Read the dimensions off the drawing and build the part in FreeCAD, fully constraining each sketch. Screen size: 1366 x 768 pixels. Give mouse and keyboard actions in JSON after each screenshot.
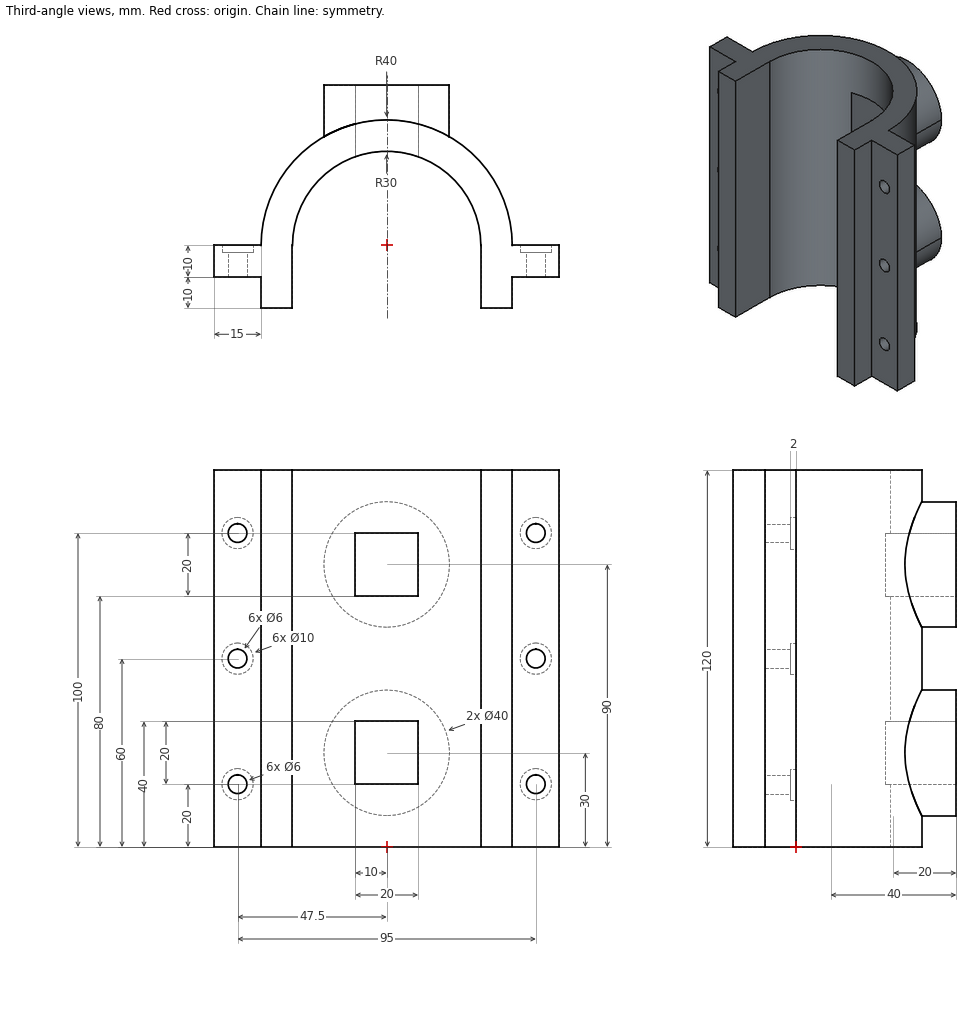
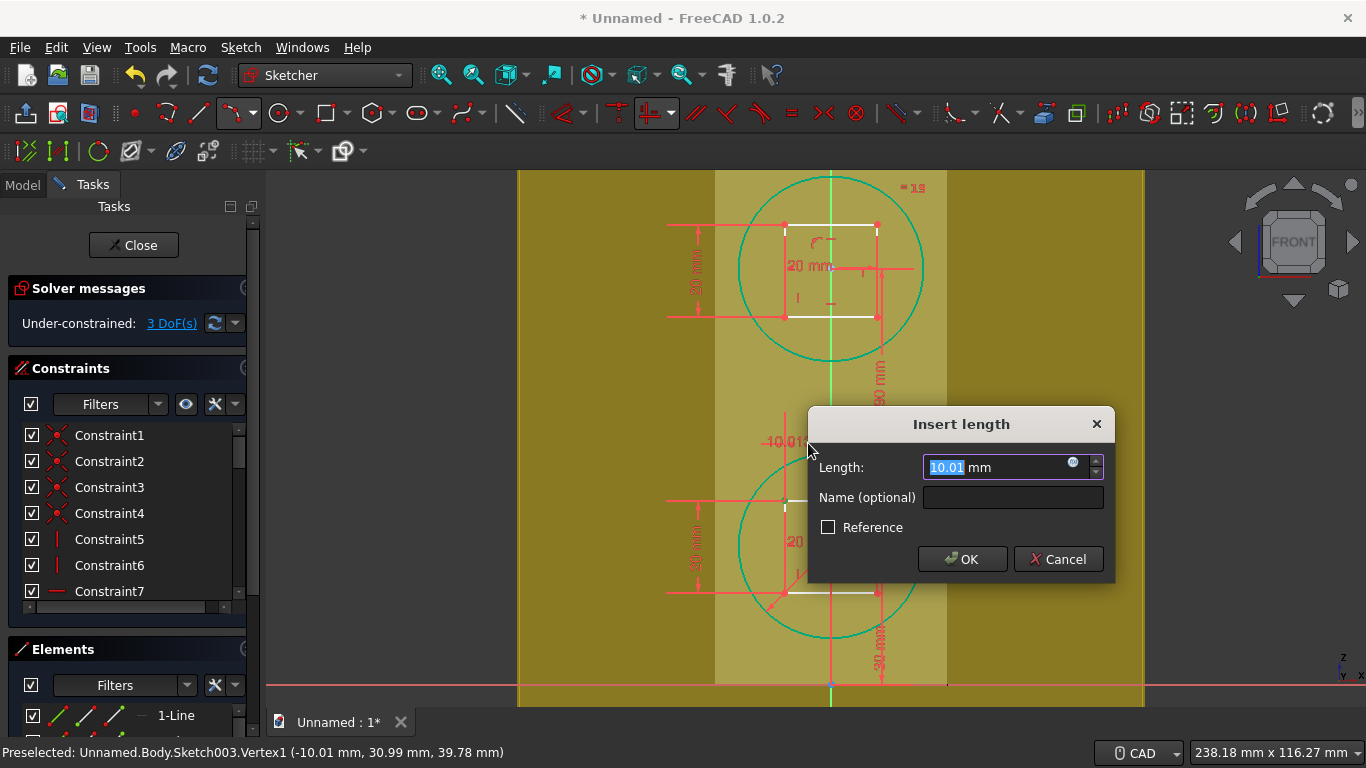
{"action": "type", "text": "10"}
{"action": "key", "text": "Return"}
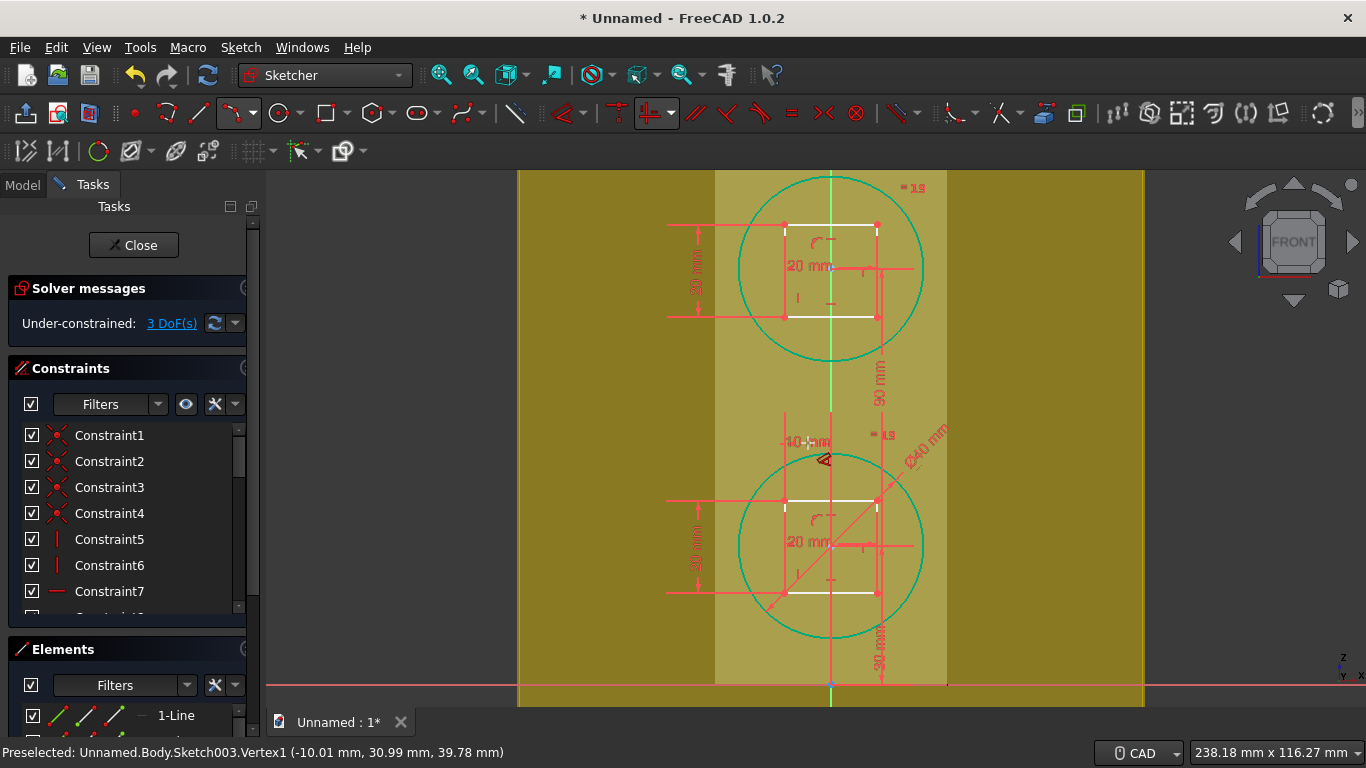
{"action": "left_click", "coordinate": [785, 501]}
{"action": "left_click", "coordinate": [751, 631]}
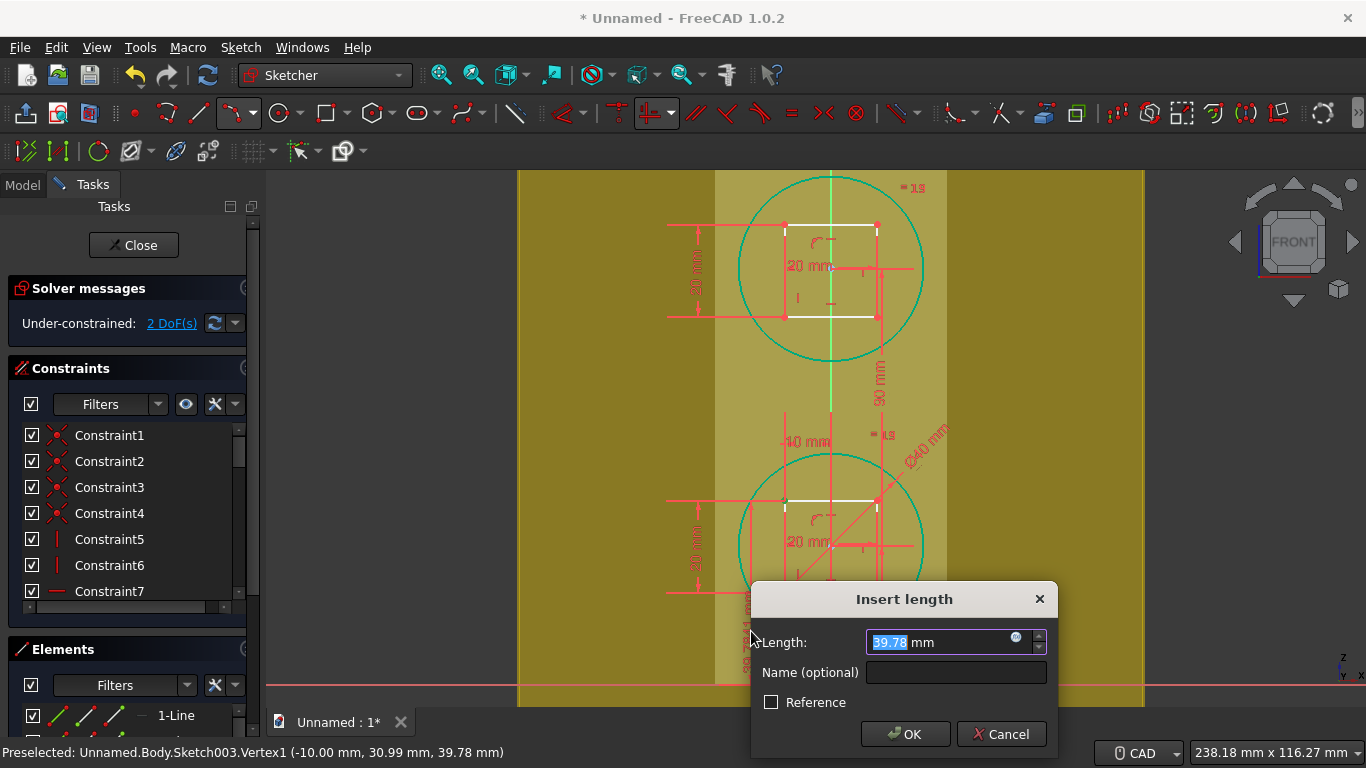
{"action": "type", "text": "40"}
{"action": "key", "text": "Return"}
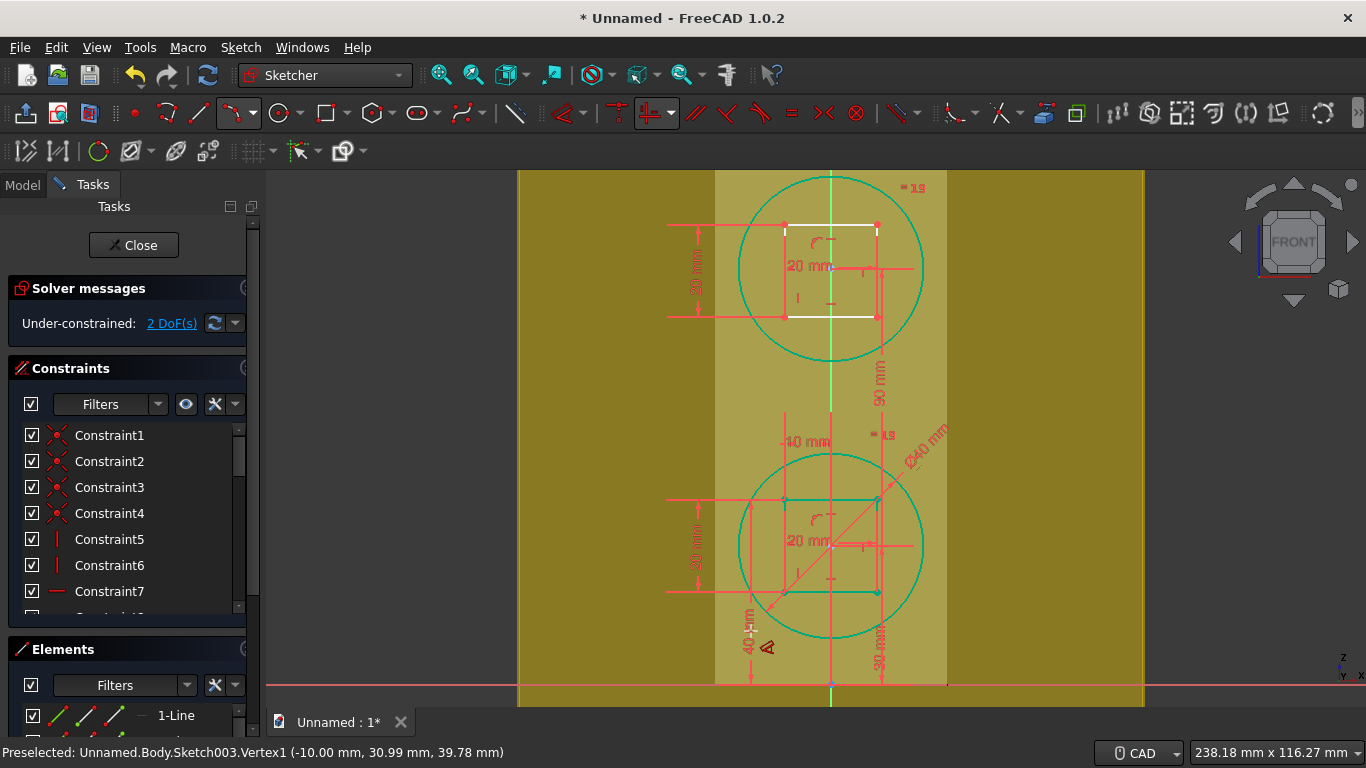
{"action": "left_click", "coordinate": [785, 225]}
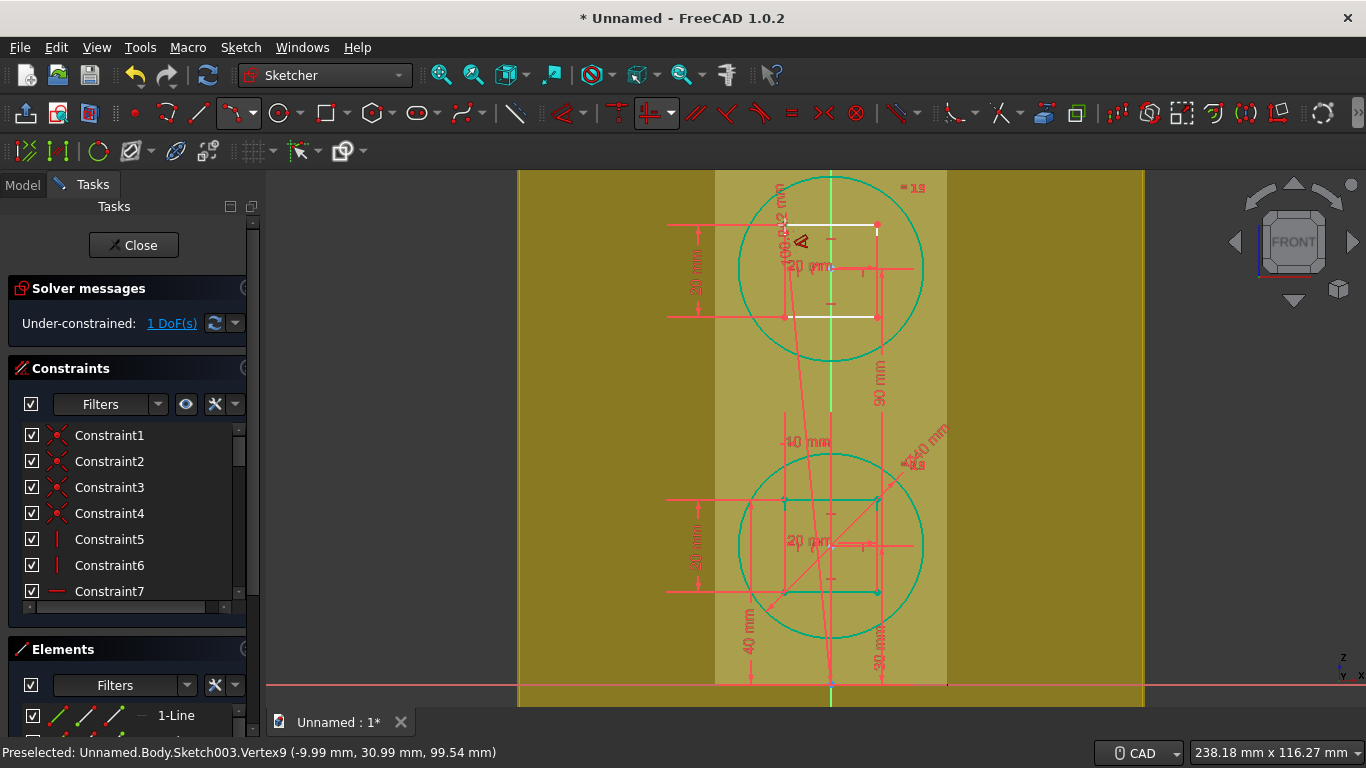
{"action": "key", "text": "Escape"}
{"action": "key", "text": "Escape"}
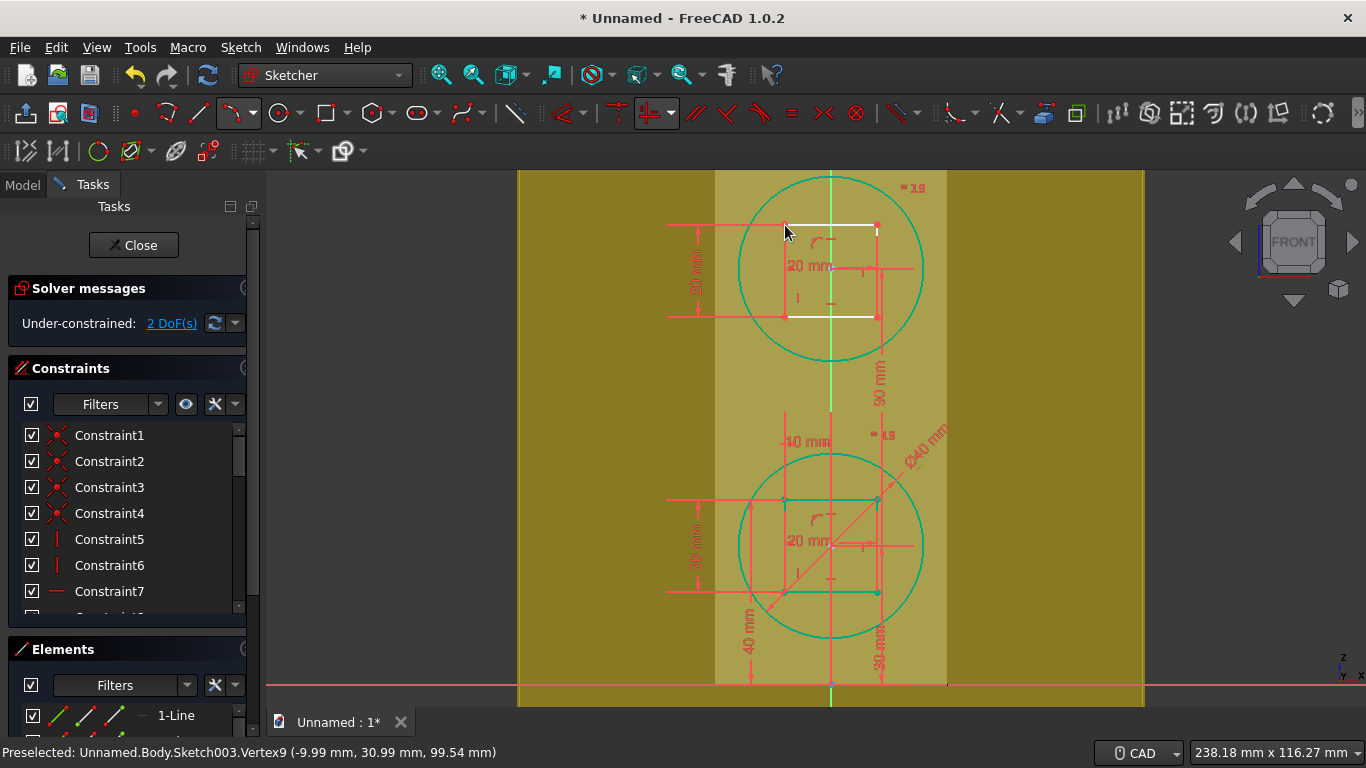
{"action": "left_click", "coordinate": [785, 225]}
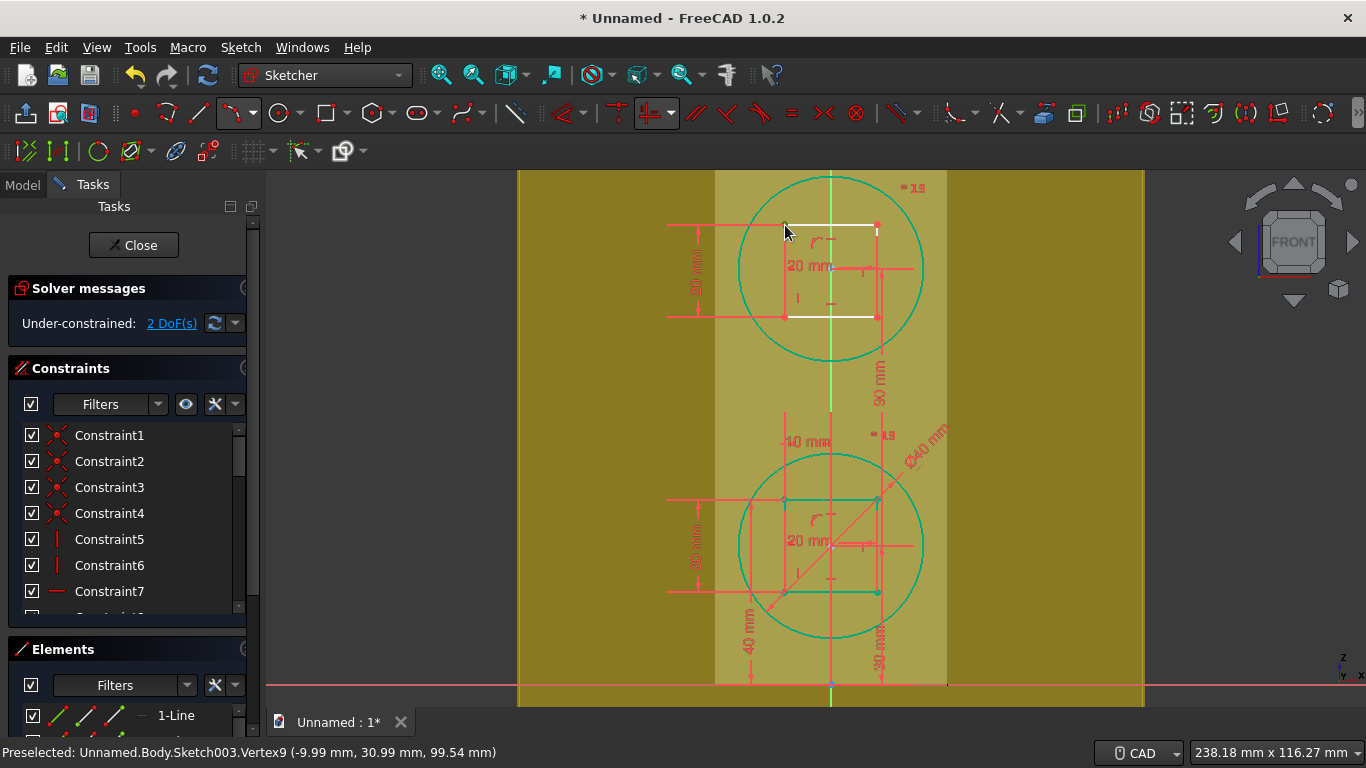
{"action": "key", "text": "l"}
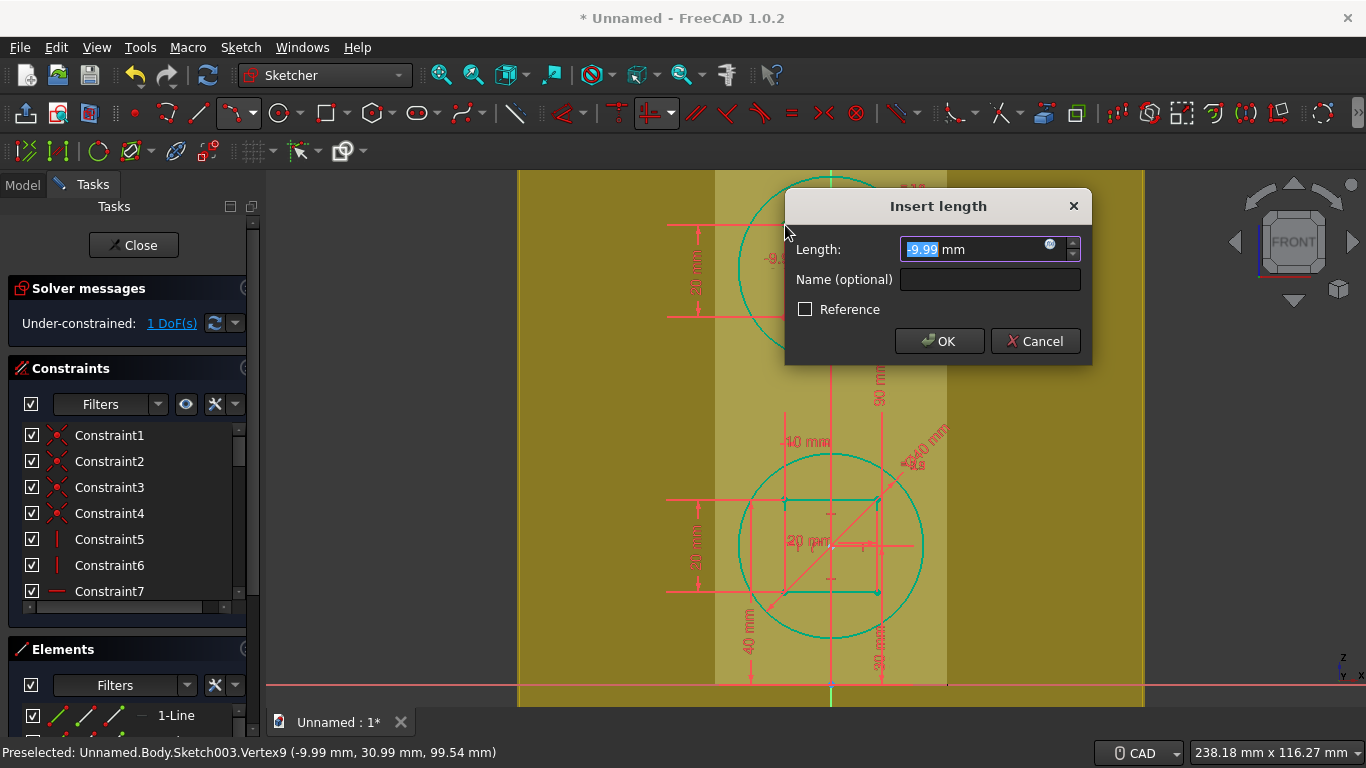
{"action": "type", "text": "-10"}
{"action": "key", "text": "Return"}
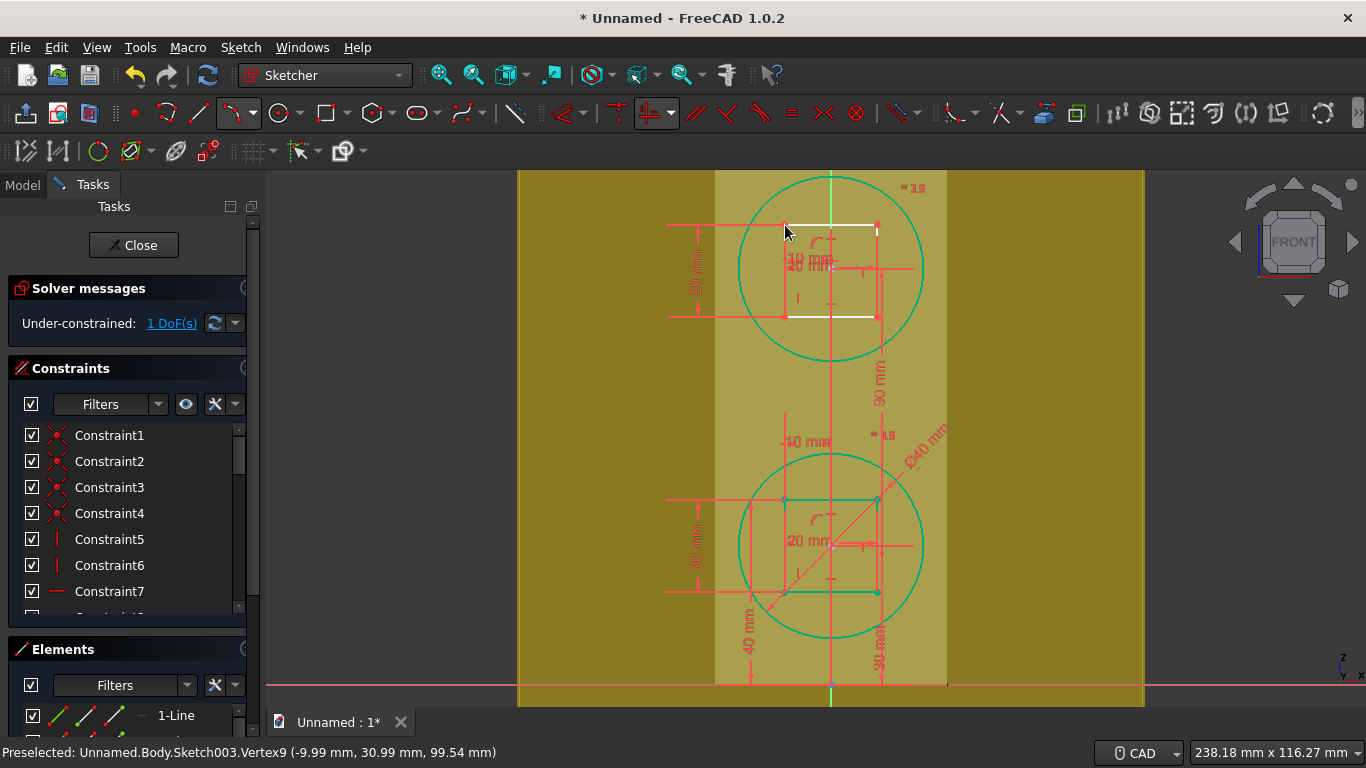
{"action": "left_click", "coordinate": [785, 317]}